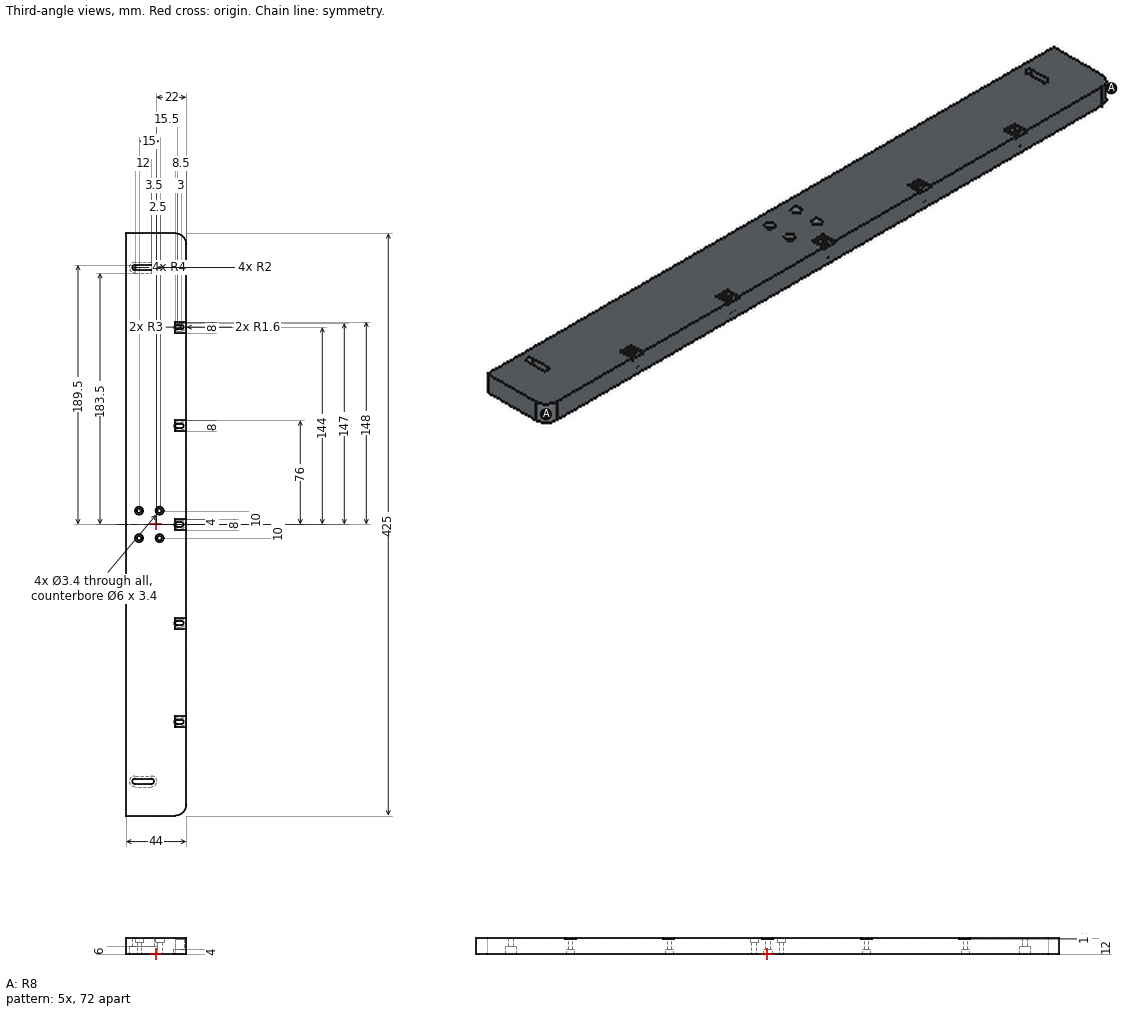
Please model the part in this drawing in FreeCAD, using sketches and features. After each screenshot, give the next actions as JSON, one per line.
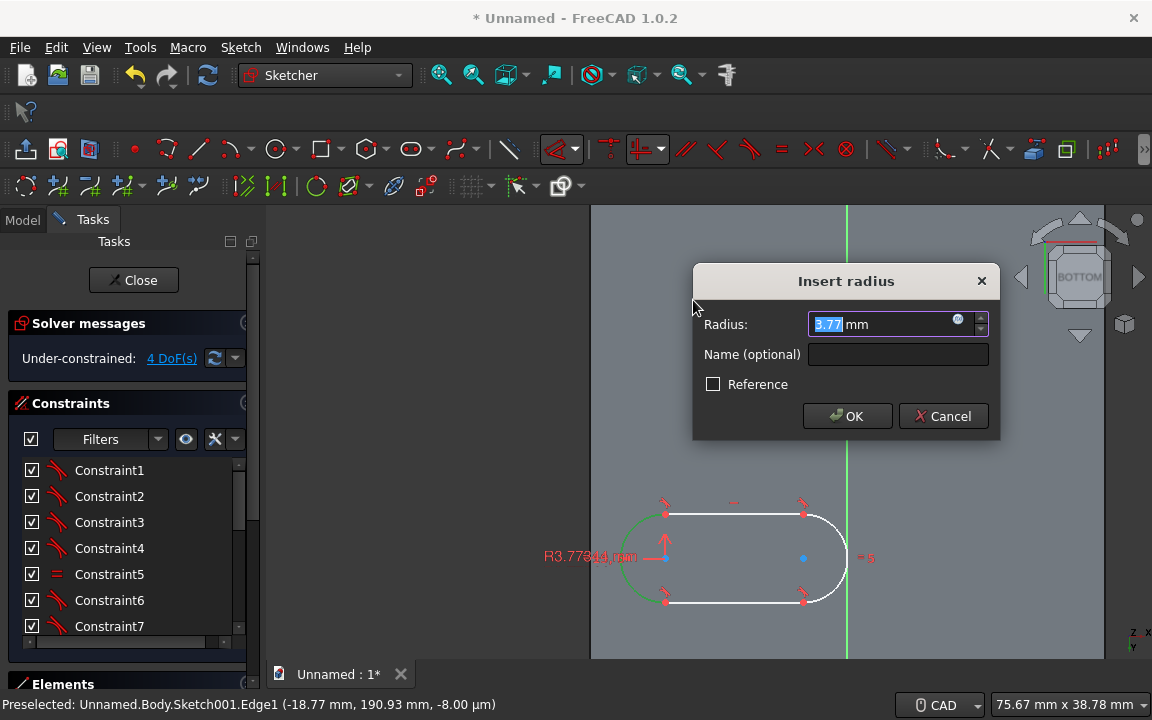
{"action": "type", "text": "4"}
{"action": "key", "text": "Return"}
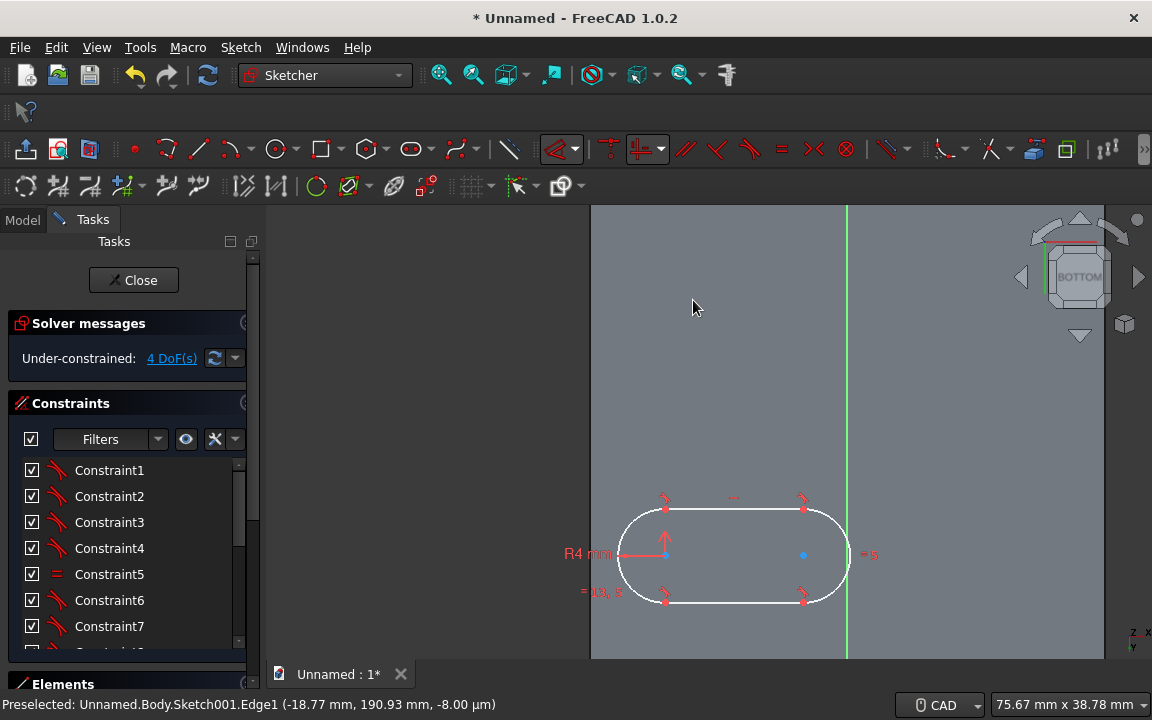
{"action": "scroll", "coordinate": [634, 567], "scroll_direction": "down", "scroll_amount": 14}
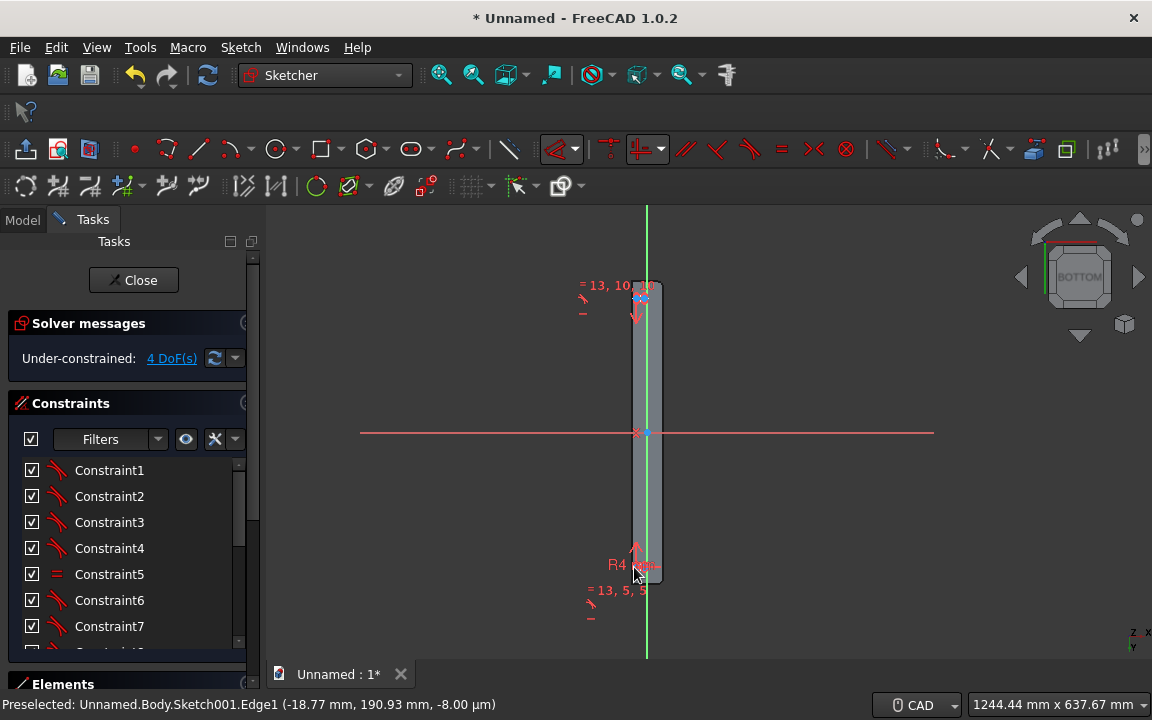
{"action": "scroll", "coordinate": [639, 564], "scroll_direction": "up", "scroll_amount": 9}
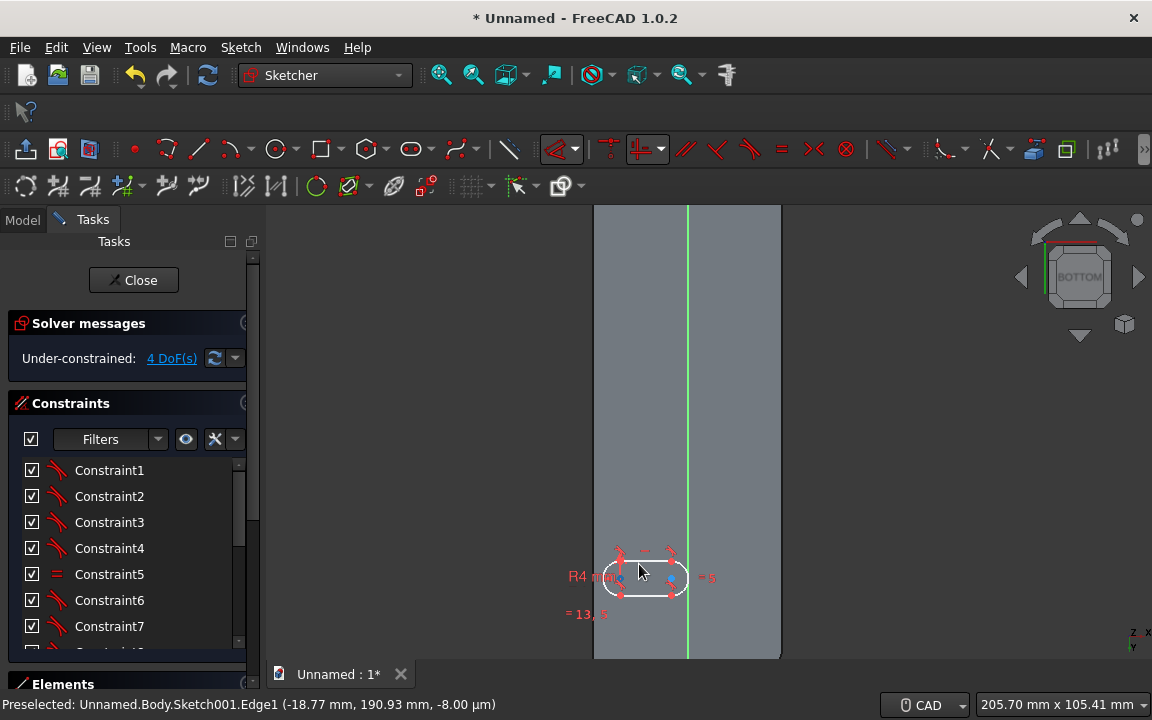
{"action": "left_click", "coordinate": [636, 561]}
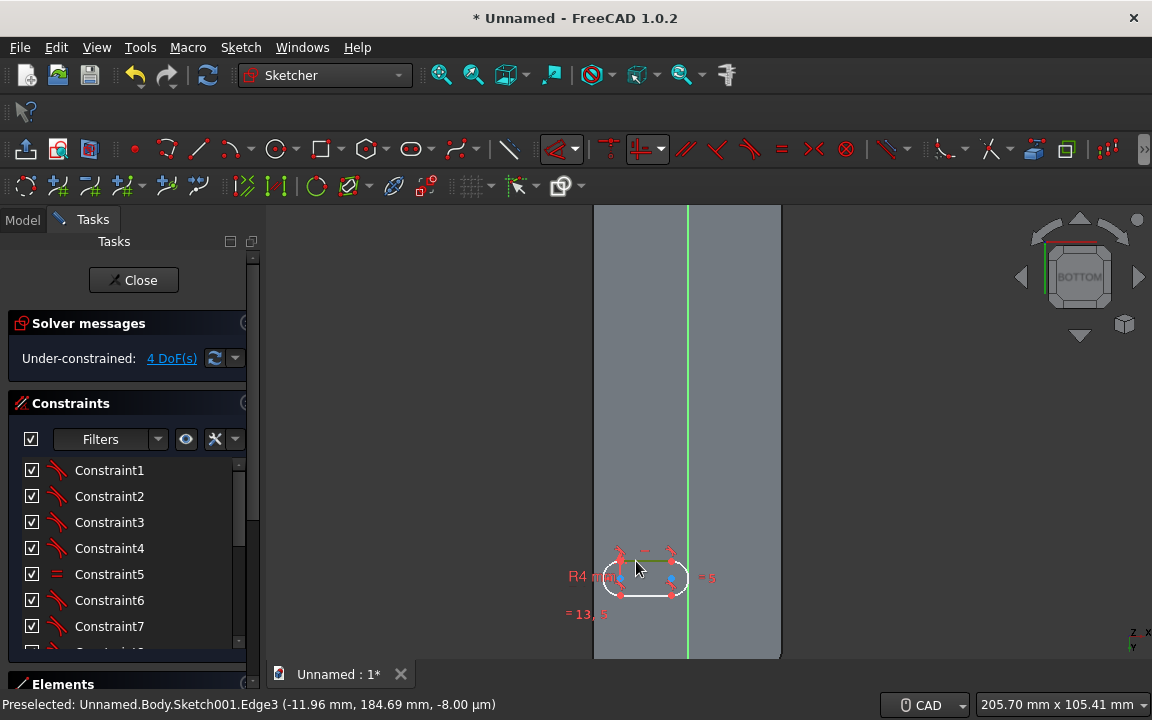
{"action": "key", "text": "l"}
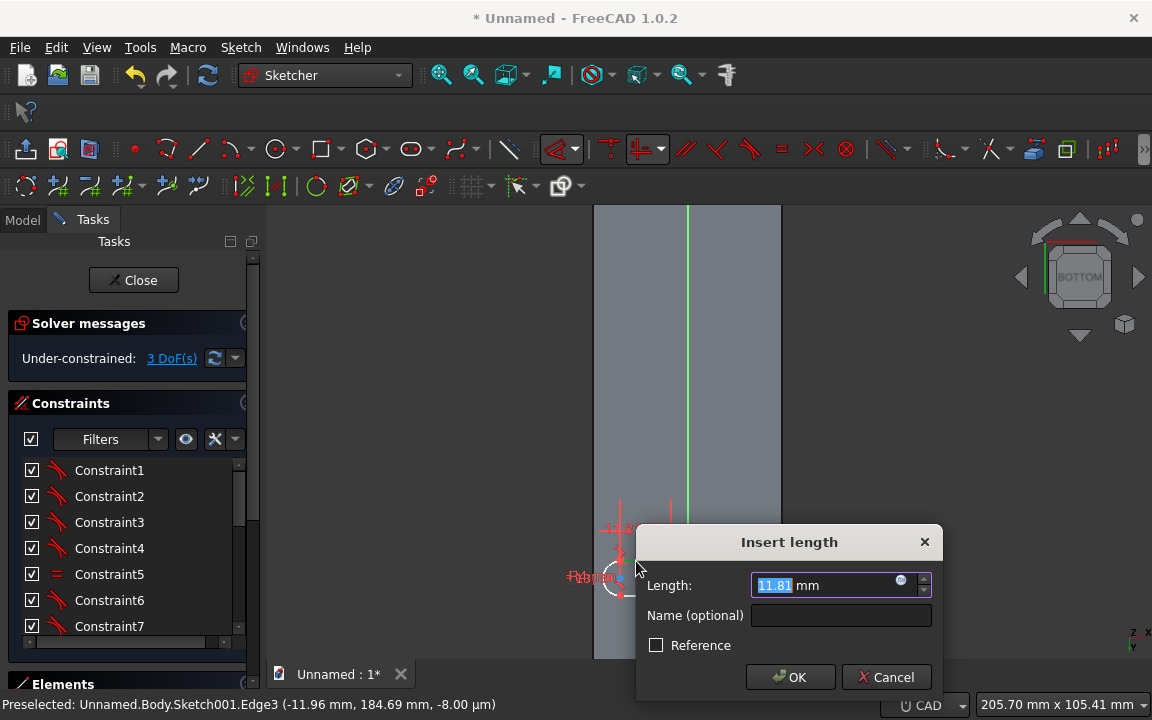
{"action": "type", "text": "12"}
{"action": "key", "text": "Return"}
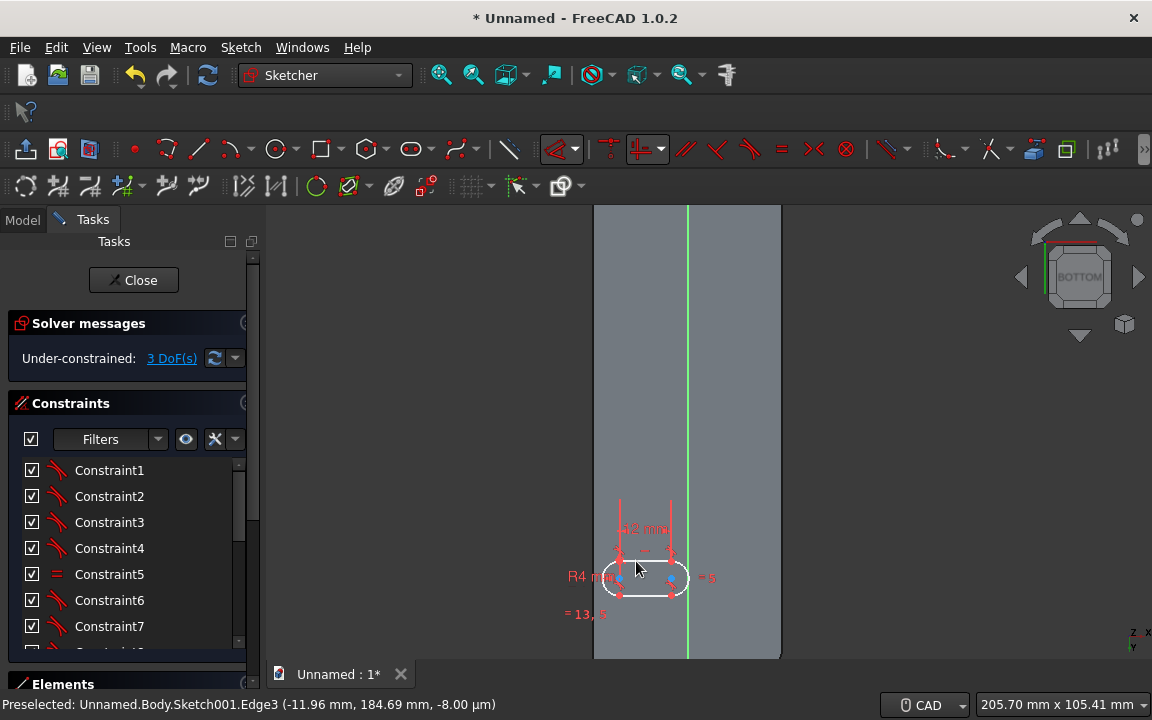
{"action": "scroll", "coordinate": [639, 564], "scroll_direction": "down", "scroll_amount": 9}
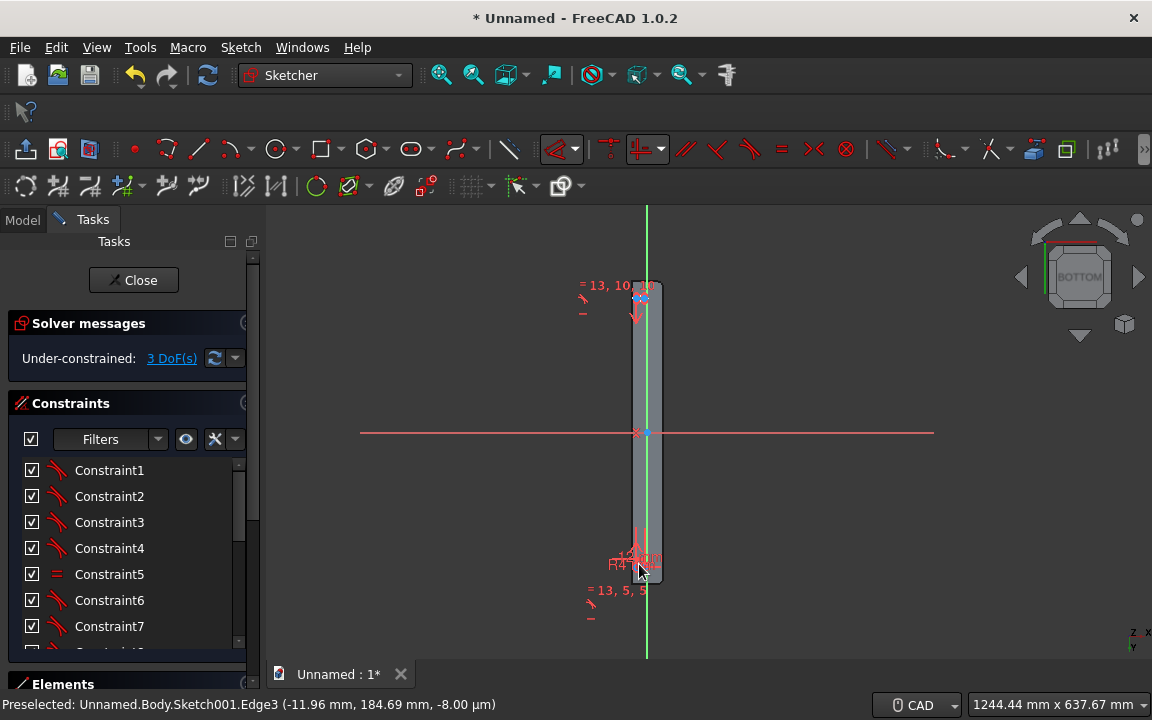
{"action": "scroll", "coordinate": [639, 296], "scroll_direction": "up", "scroll_amount": 9}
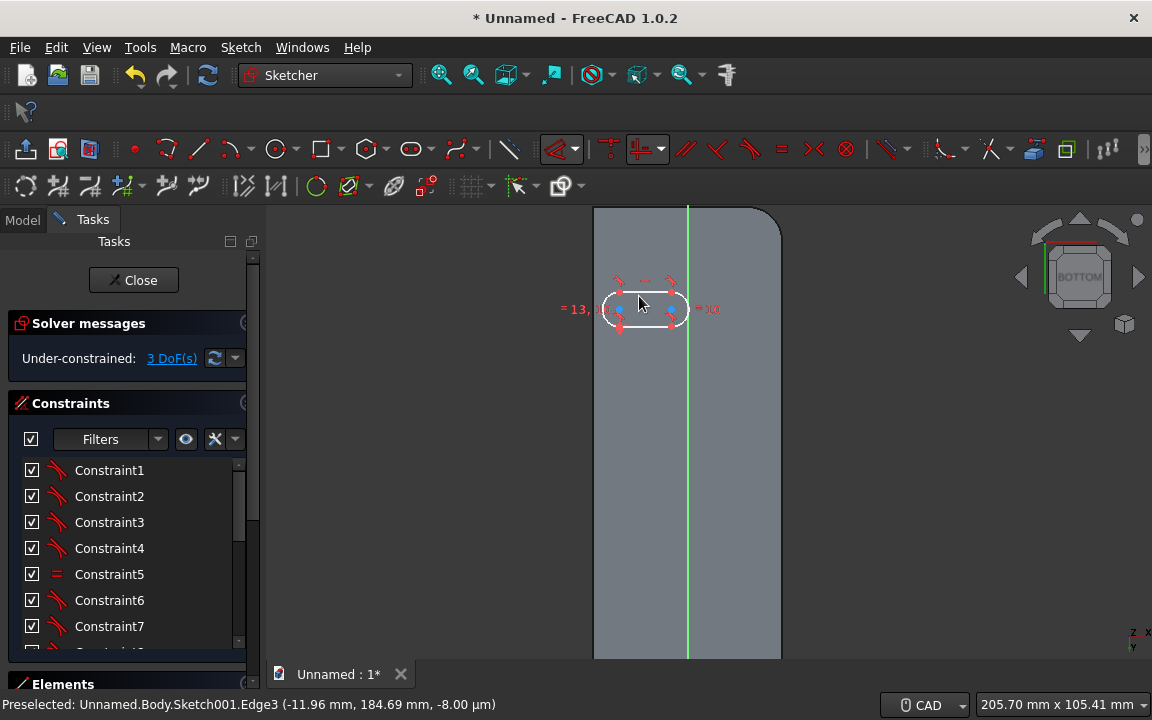
{"action": "left_click", "coordinate": [635, 292]}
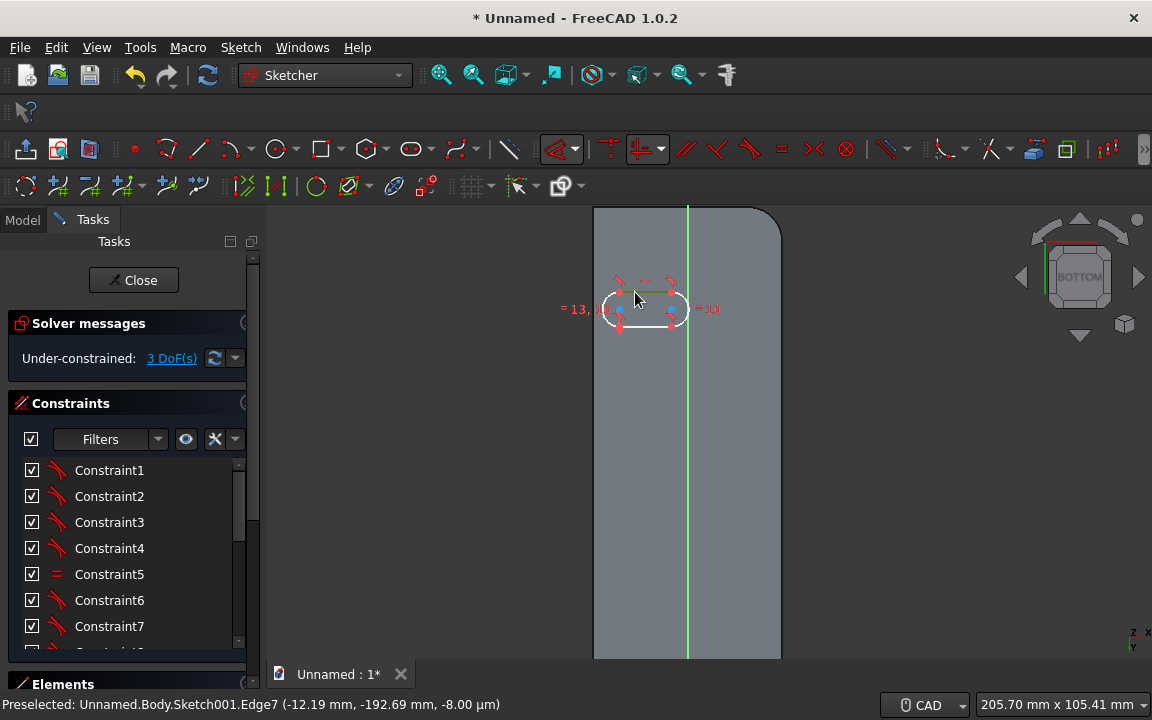
{"action": "key", "text": "l"}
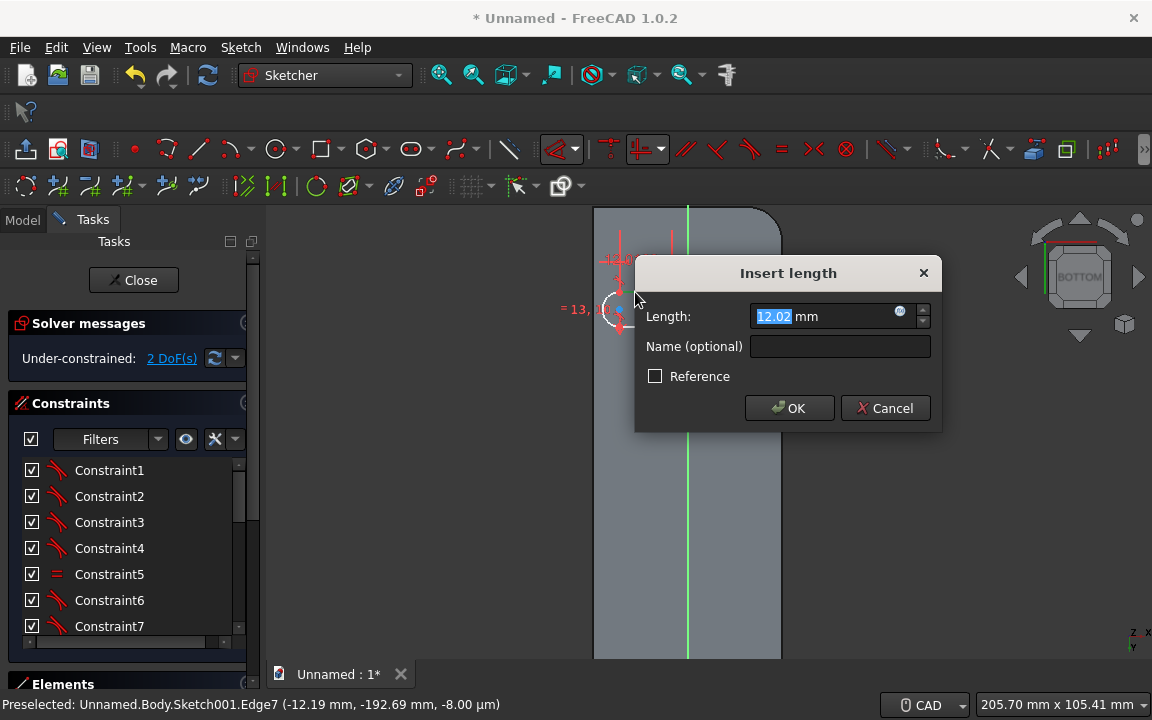
{"action": "type", "text": "12"}
{"action": "key", "text": "Return"}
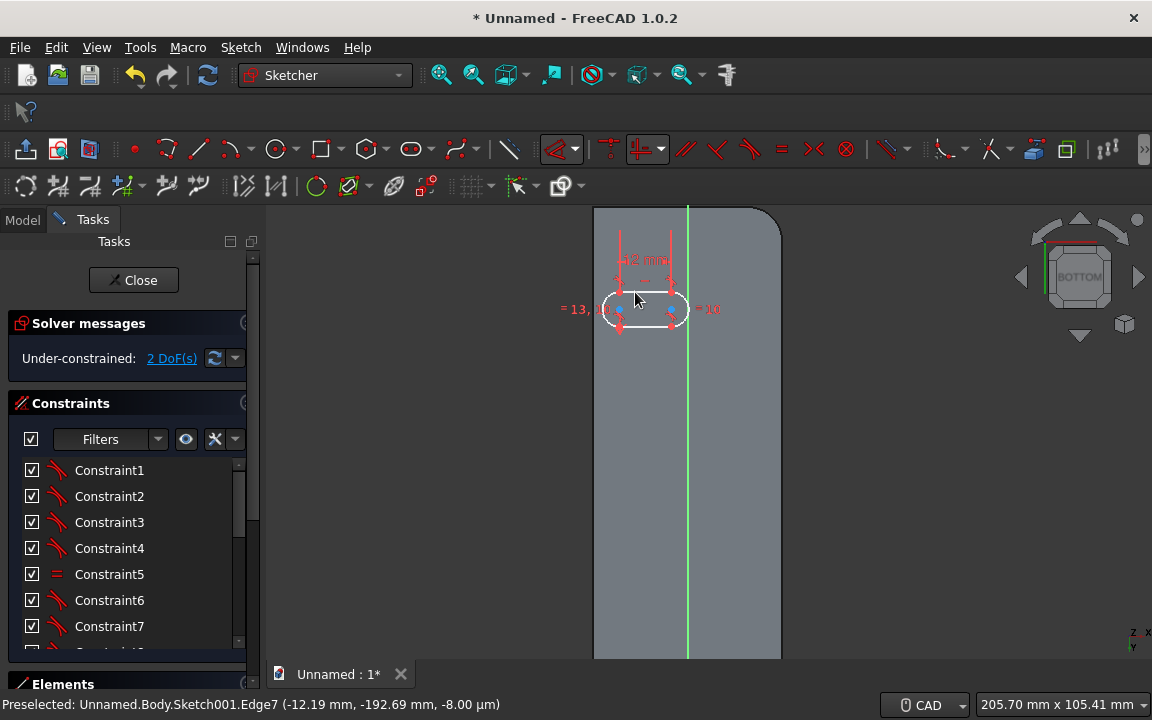
{"action": "scroll", "coordinate": [639, 295], "scroll_direction": "down", "scroll_amount": 9}